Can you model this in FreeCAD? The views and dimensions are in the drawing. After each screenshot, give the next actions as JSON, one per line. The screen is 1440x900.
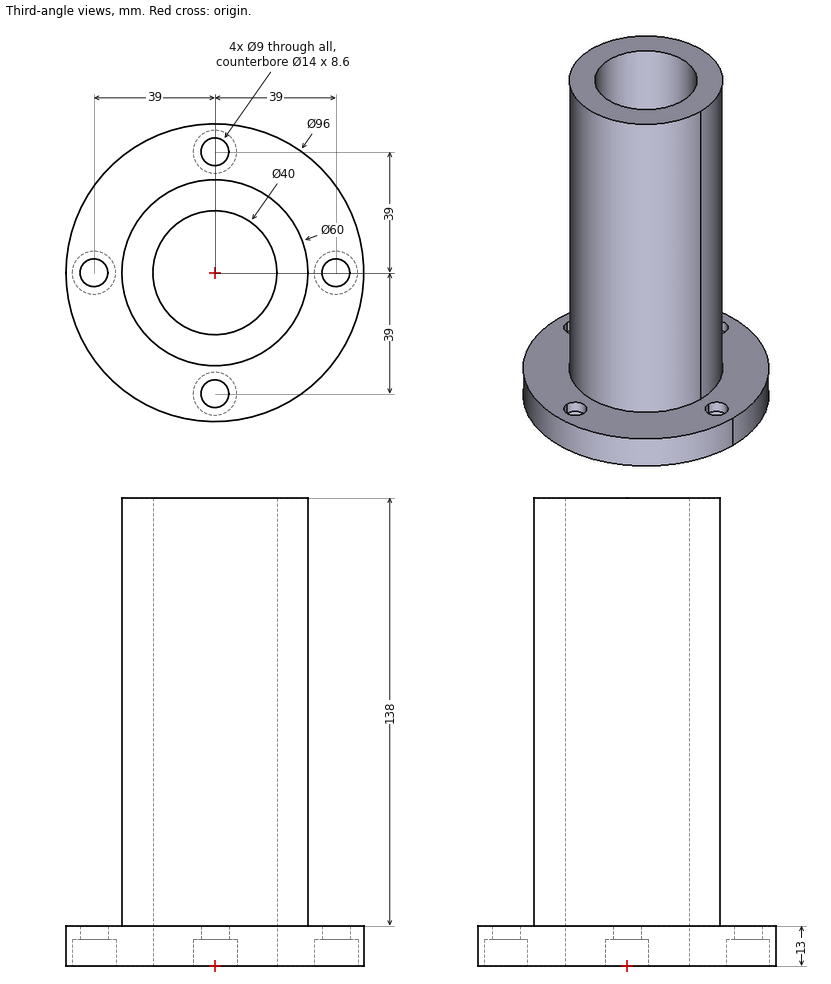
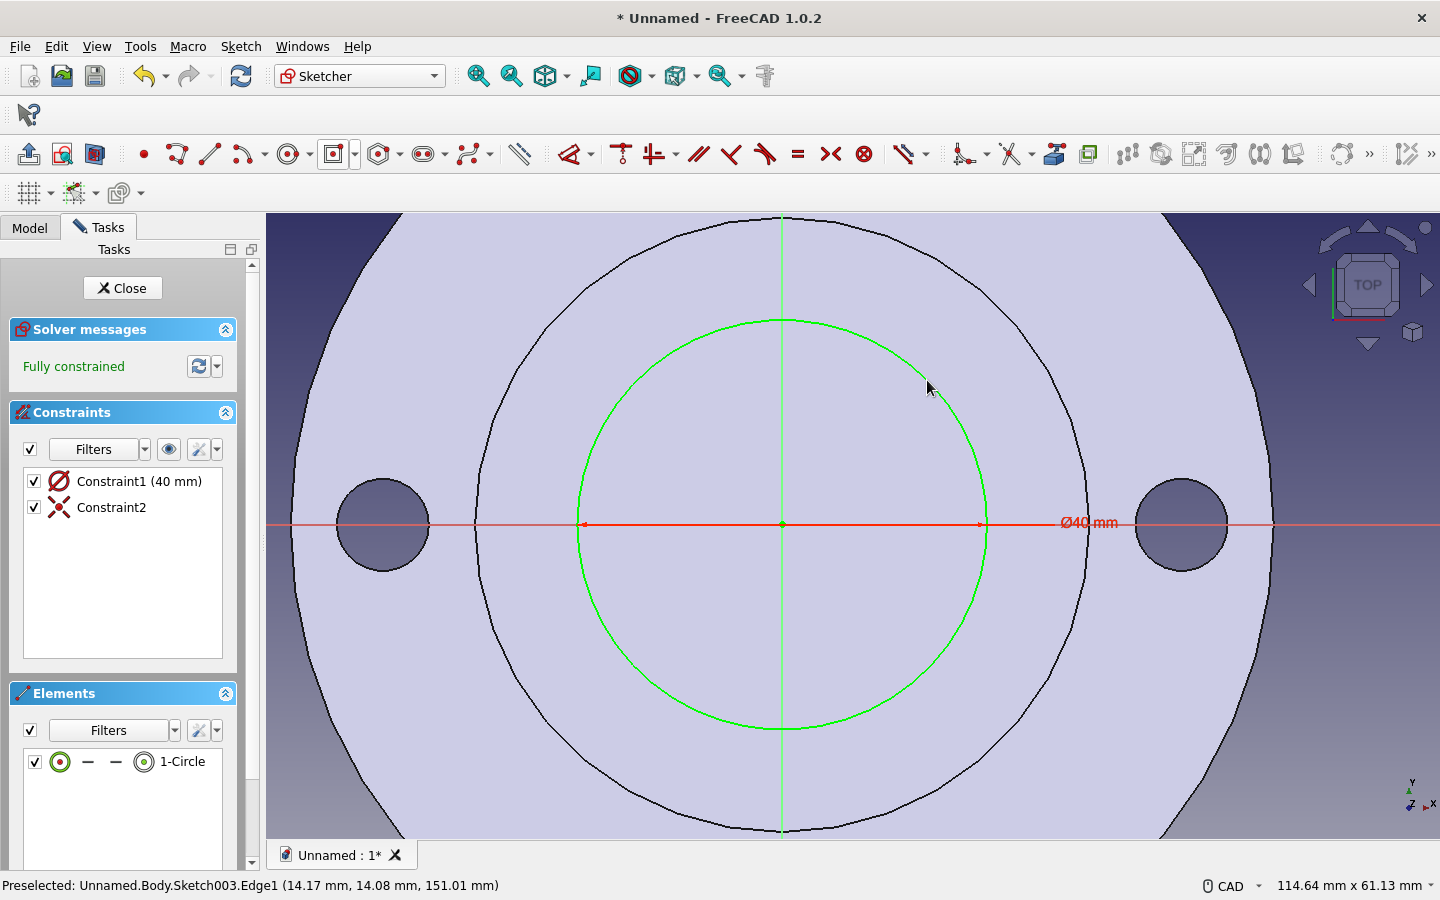
{"action": "left_click", "coordinate": [123, 288]}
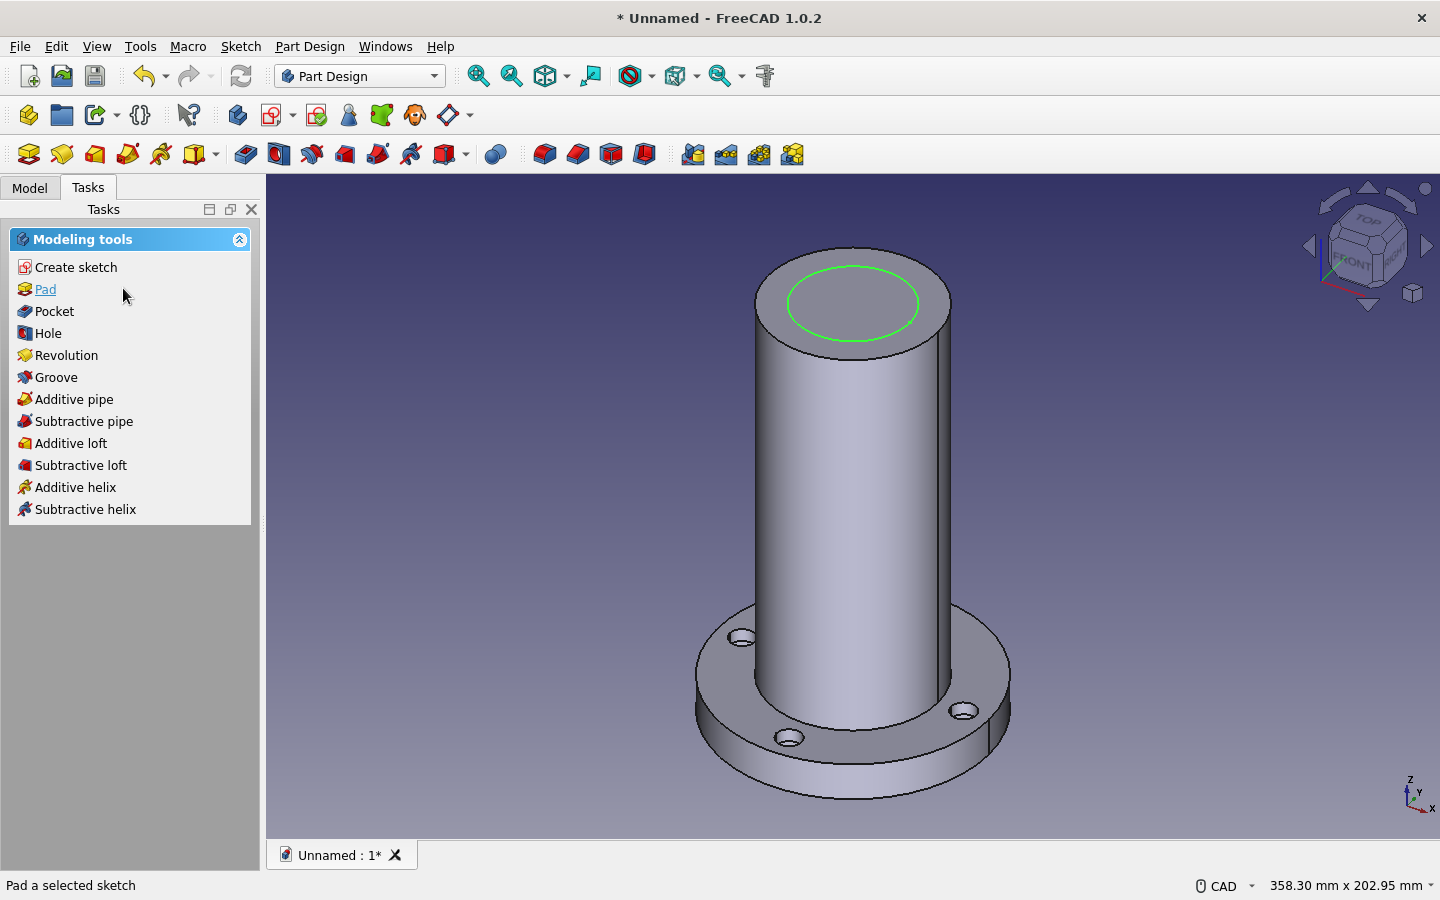
{"action": "left_click", "coordinate": [246, 154]}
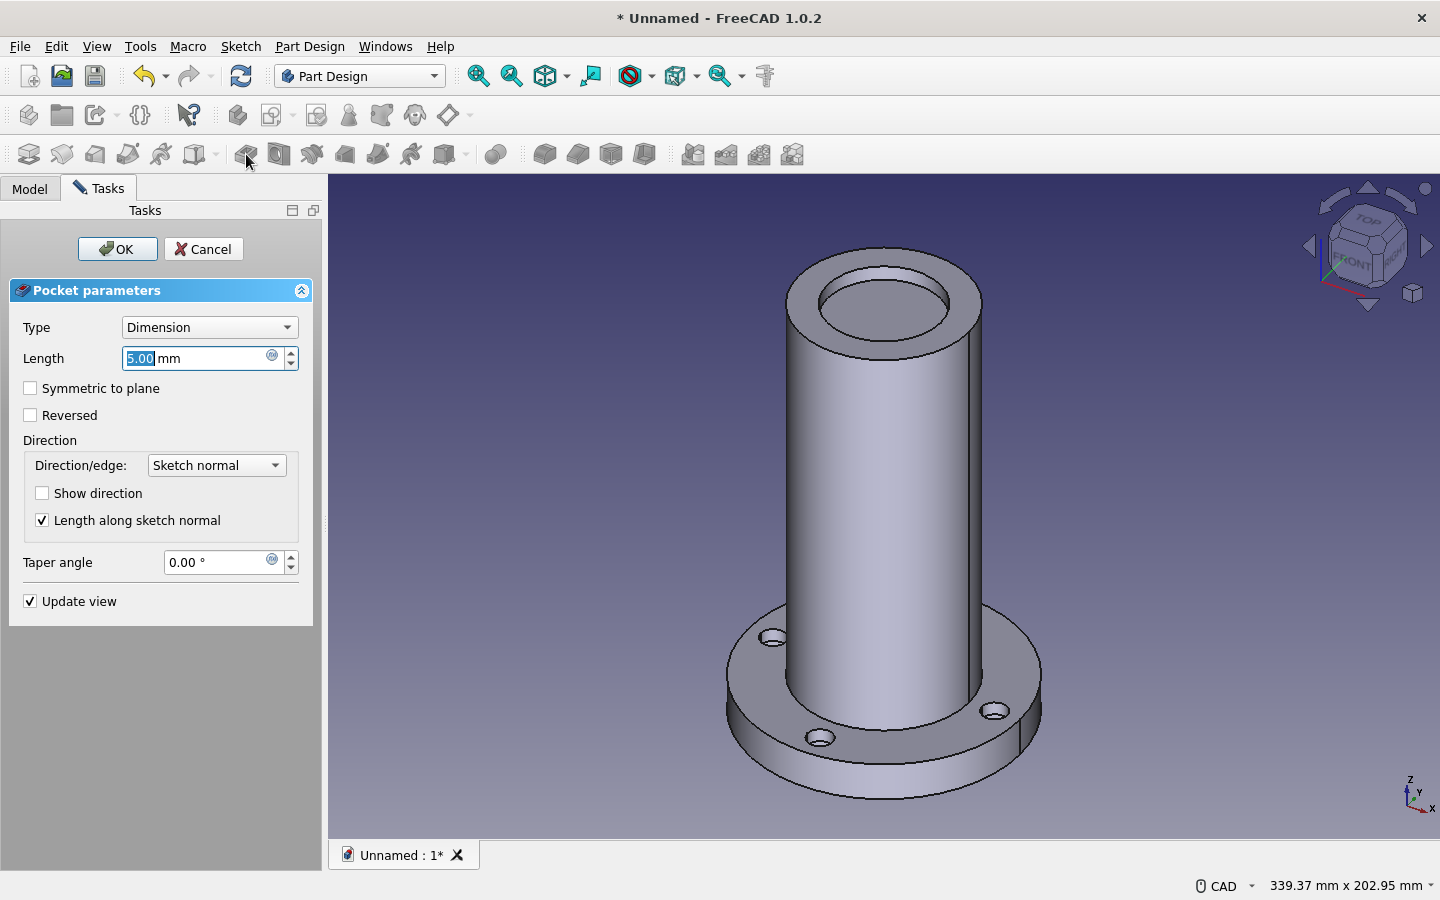
{"action": "left_click", "coordinate": [210, 328]}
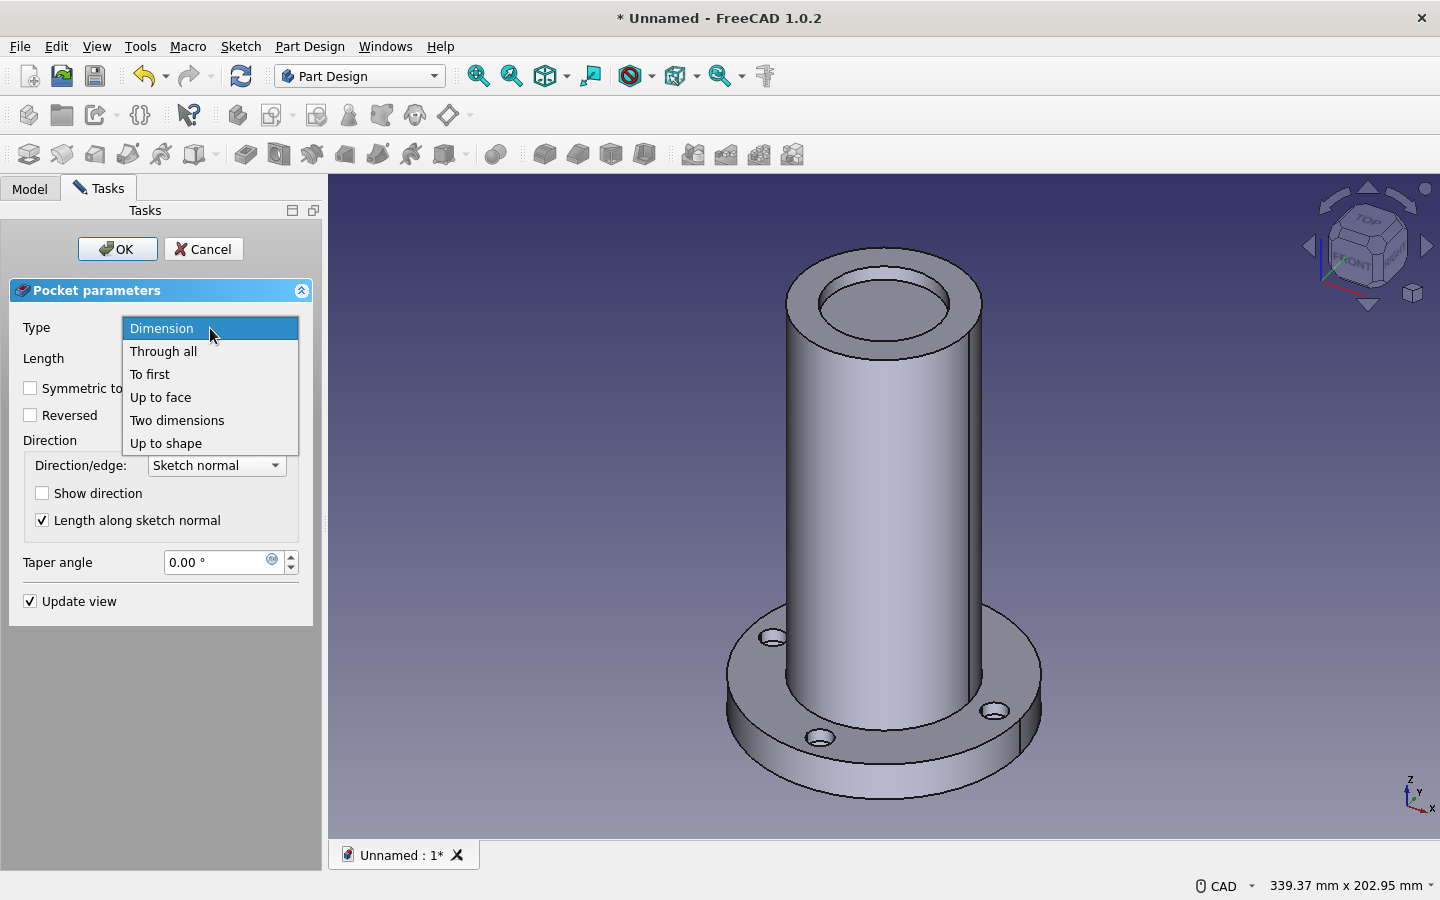
{"action": "left_click", "coordinate": [208, 352]}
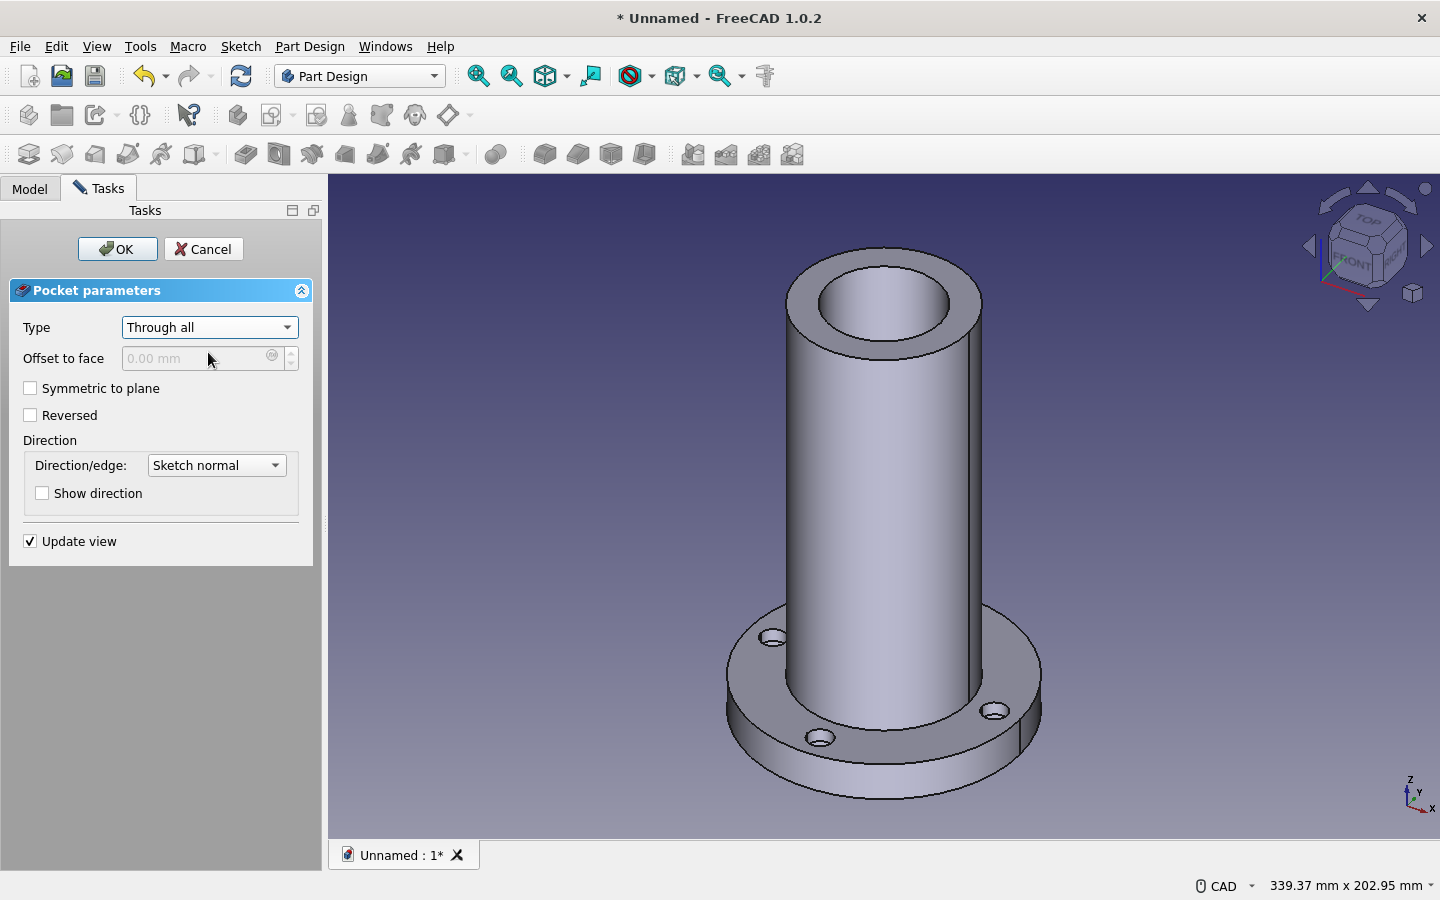
{"action": "left_click", "coordinate": [118, 249]}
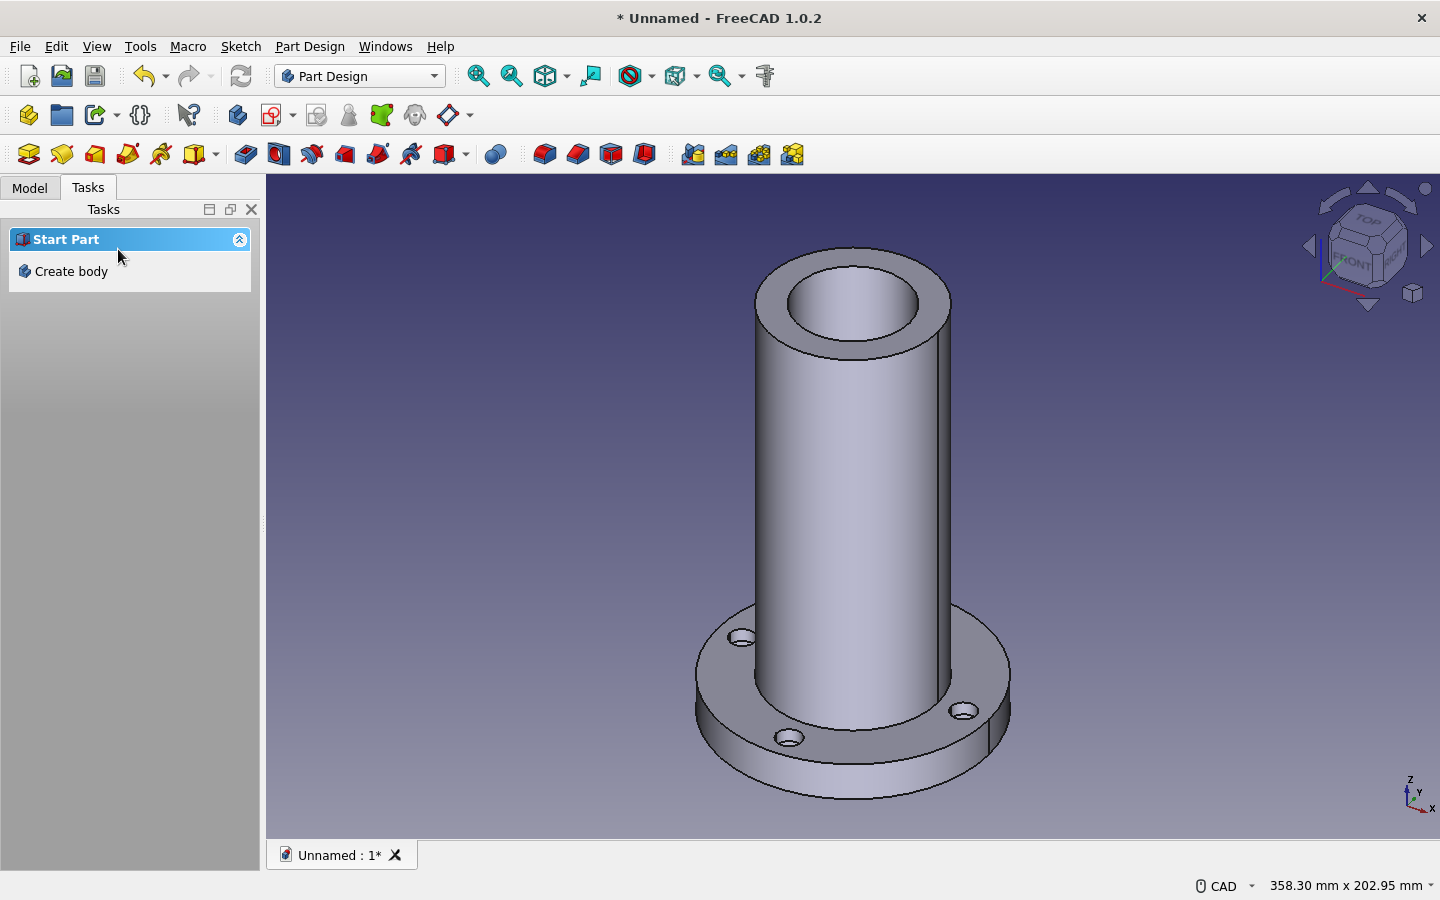
{"action": "key", "text": "0"}